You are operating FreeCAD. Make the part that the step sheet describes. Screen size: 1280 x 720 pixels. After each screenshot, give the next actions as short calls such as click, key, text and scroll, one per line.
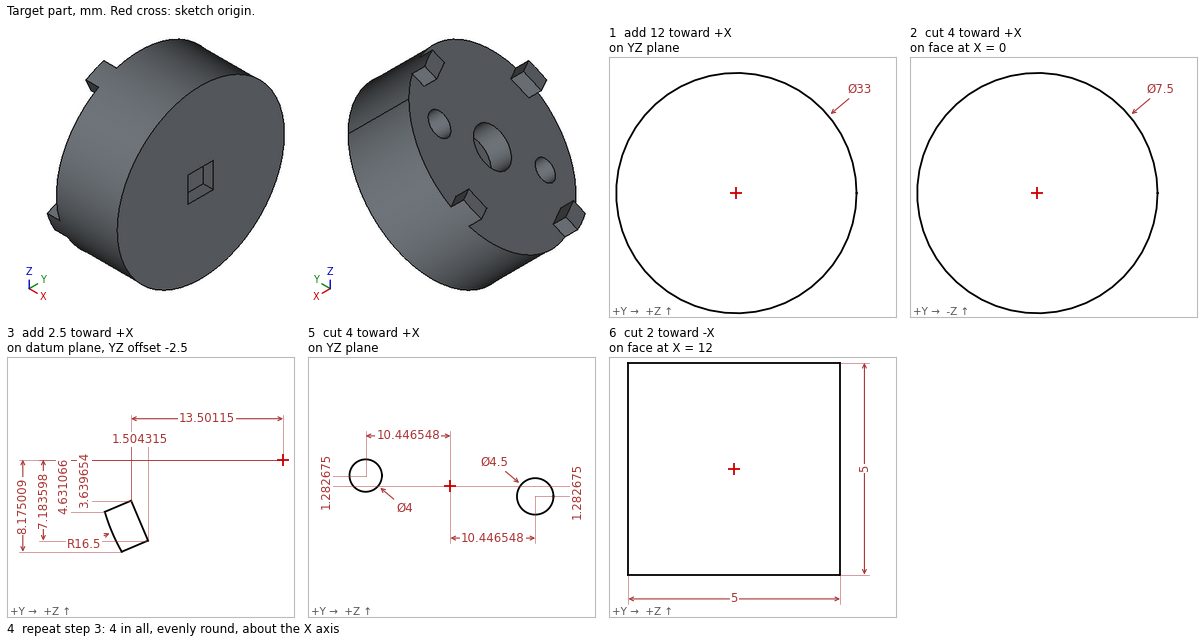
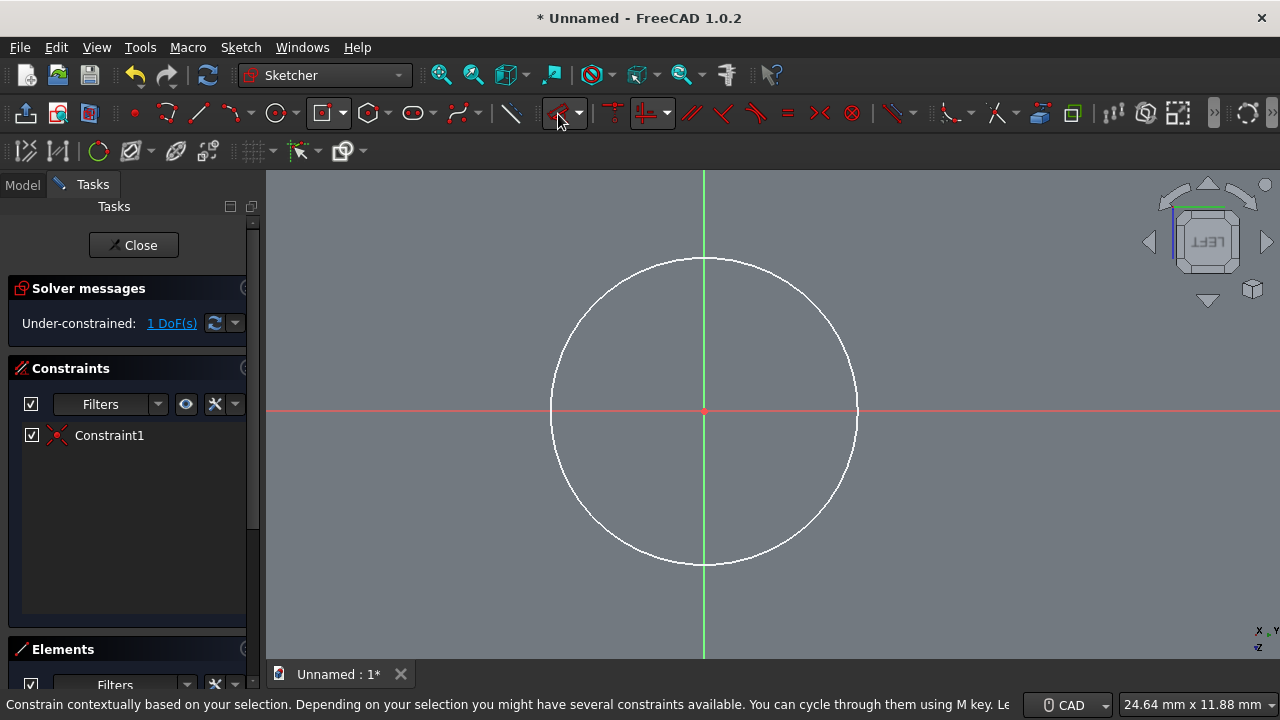
click(812, 302)
click(834, 279)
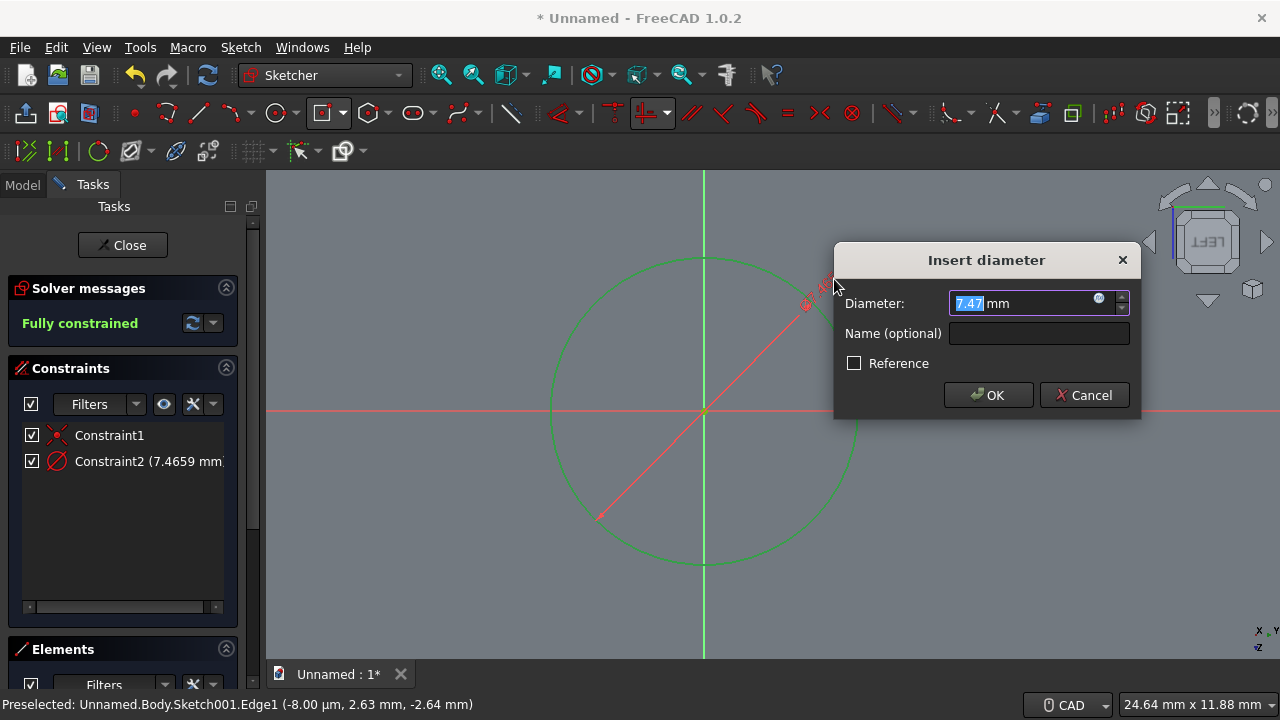
text(7.5)
key(Return)
key(Escape)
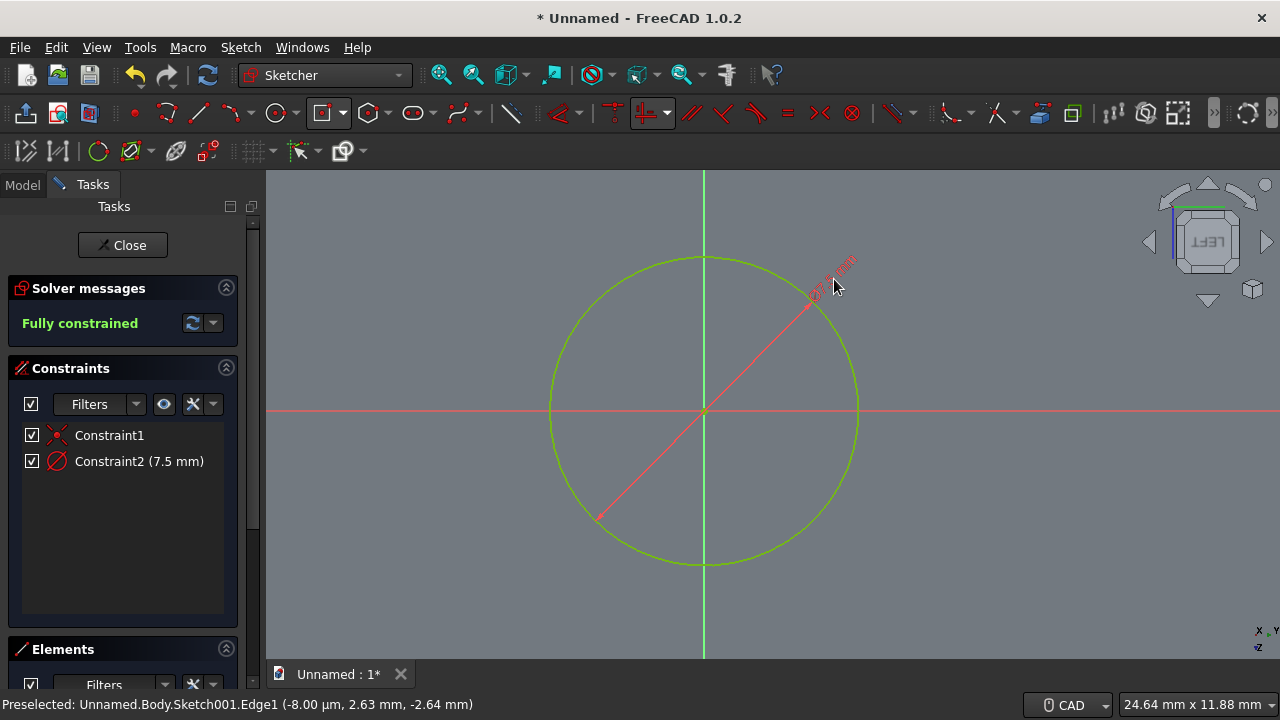
click(123, 245)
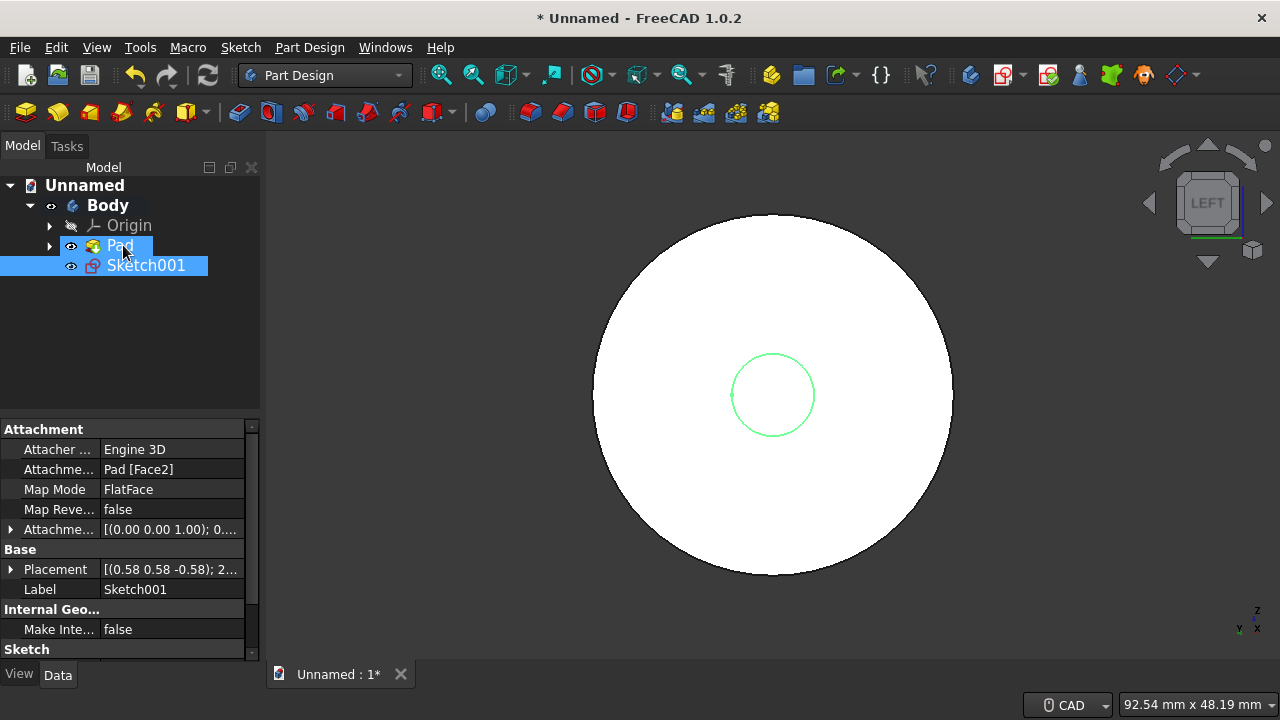
click(240, 112)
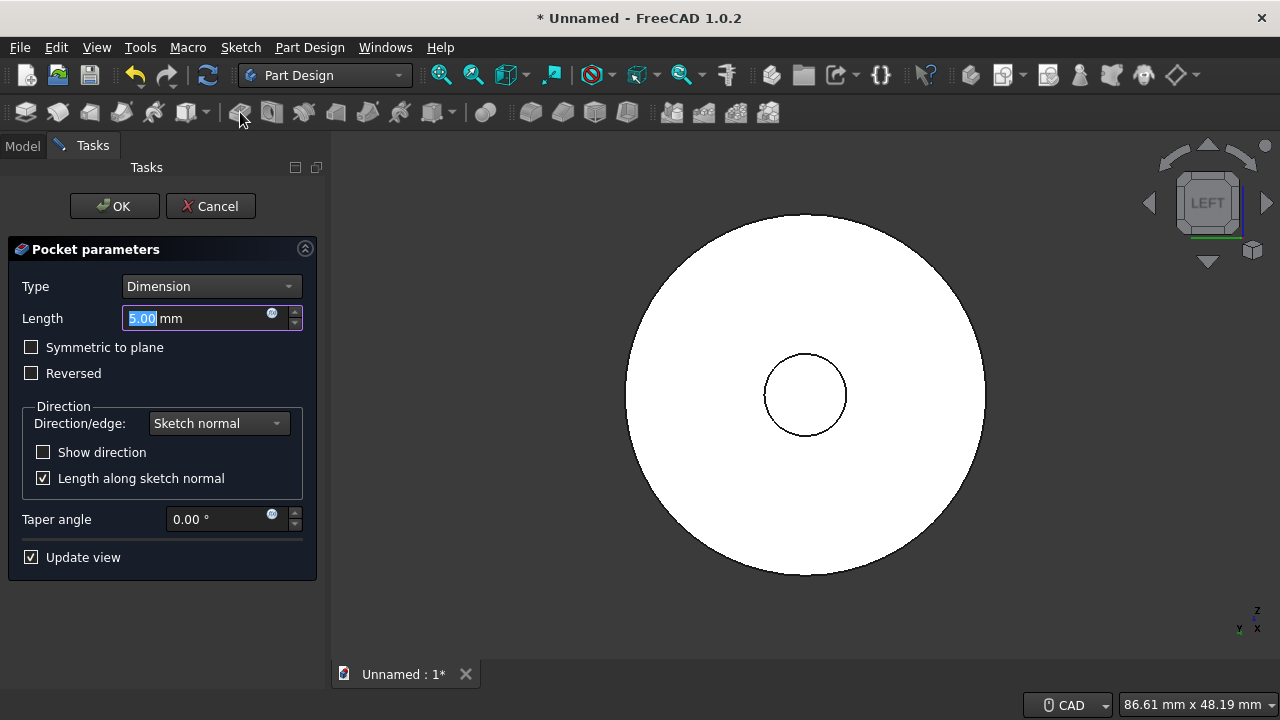
text(4)
key(Tab)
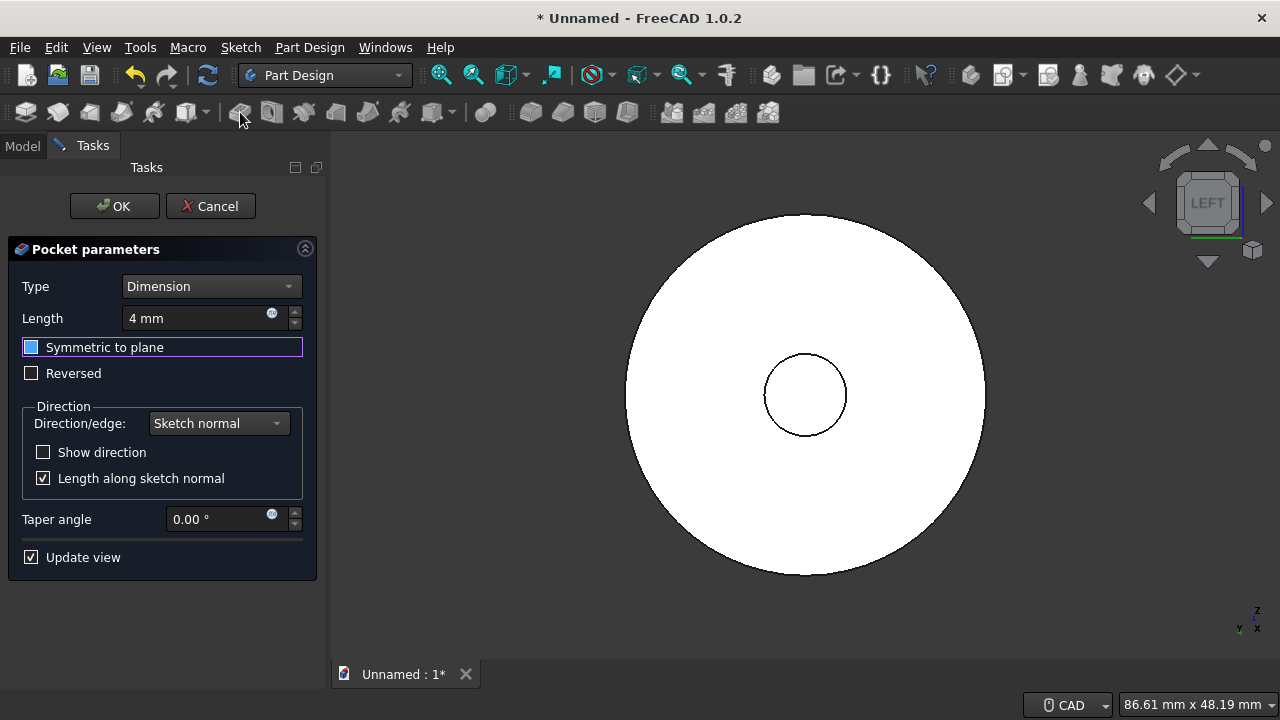
click(115, 206)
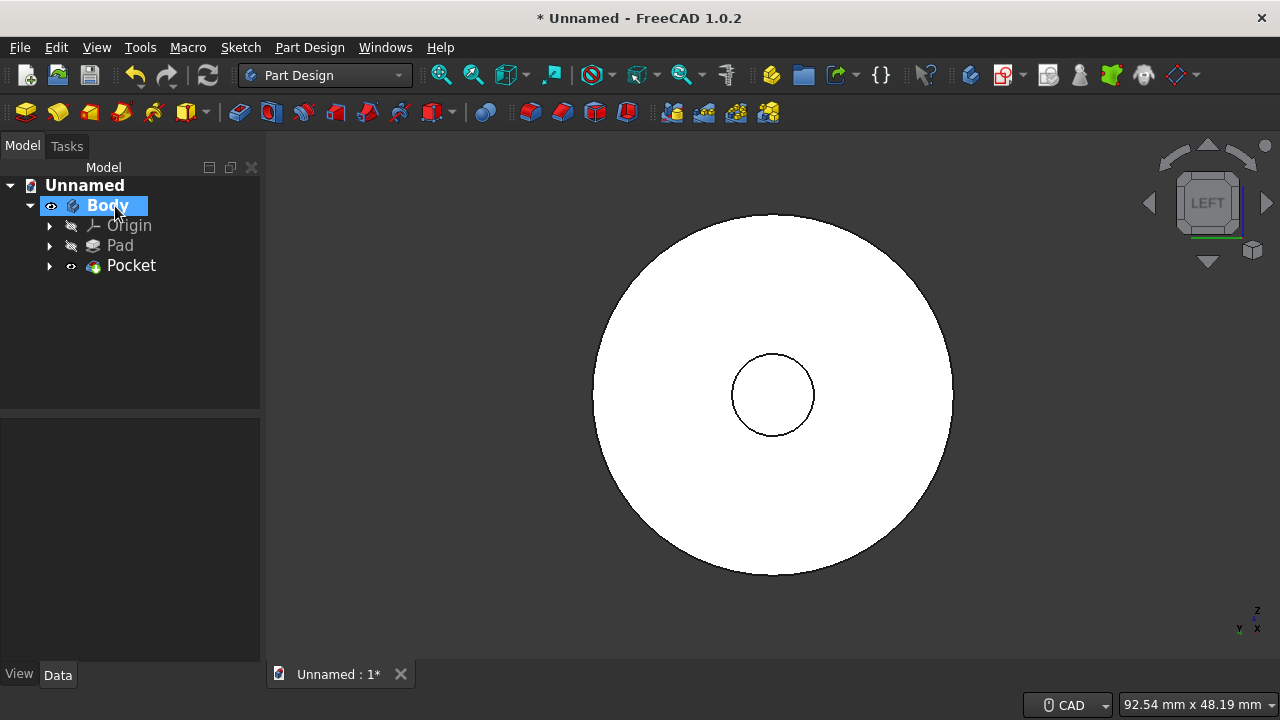
click(50, 226)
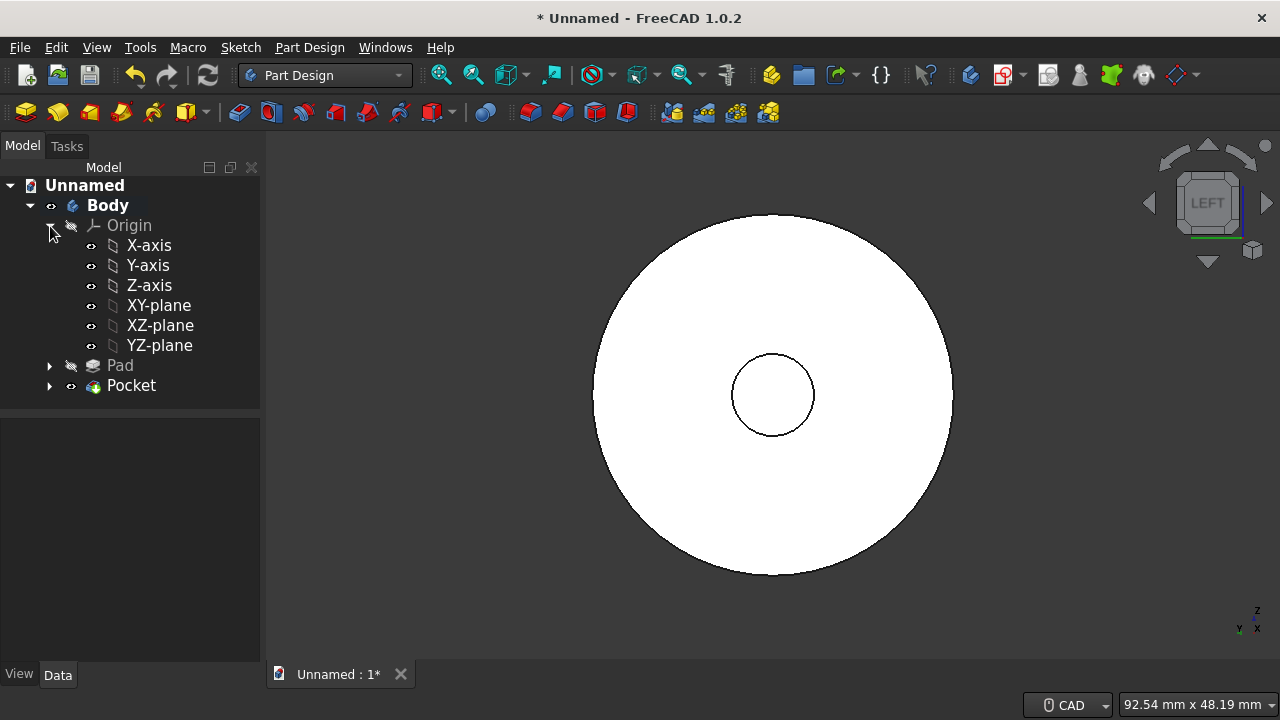
click(136, 346)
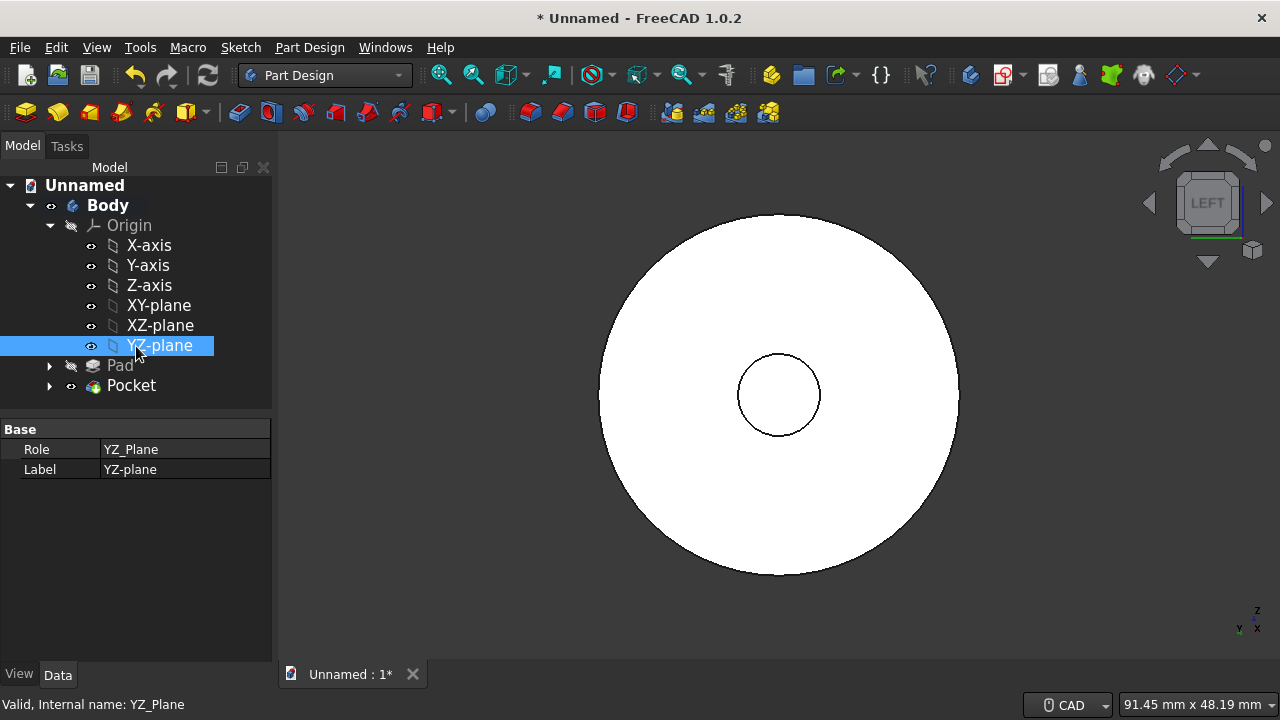
click(1176, 76)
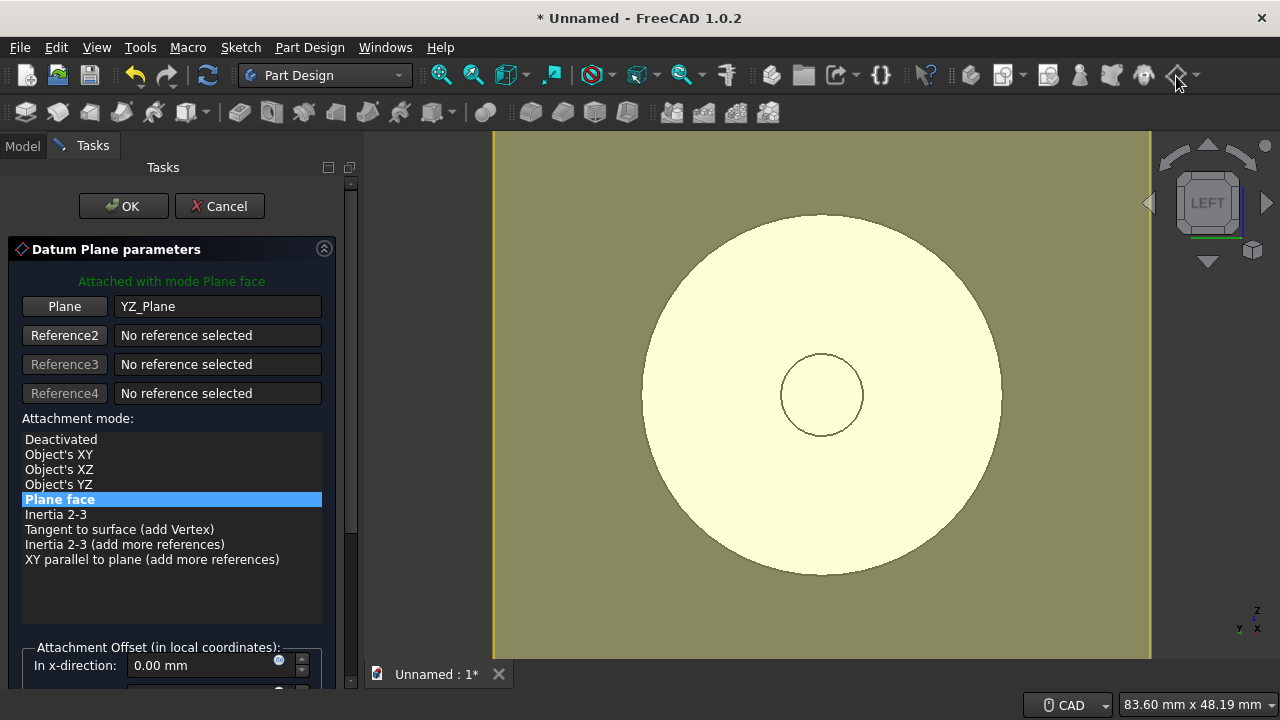
scroll(351, 432, down, 2)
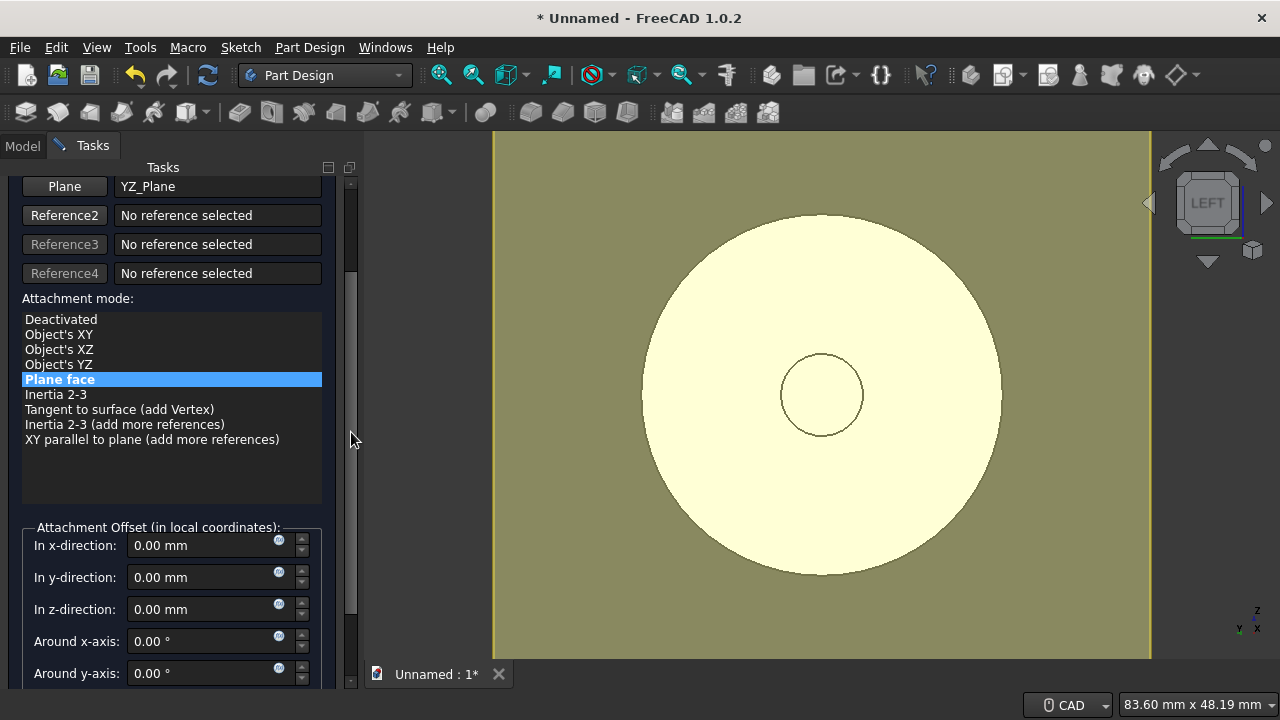
triple_click(210, 609)